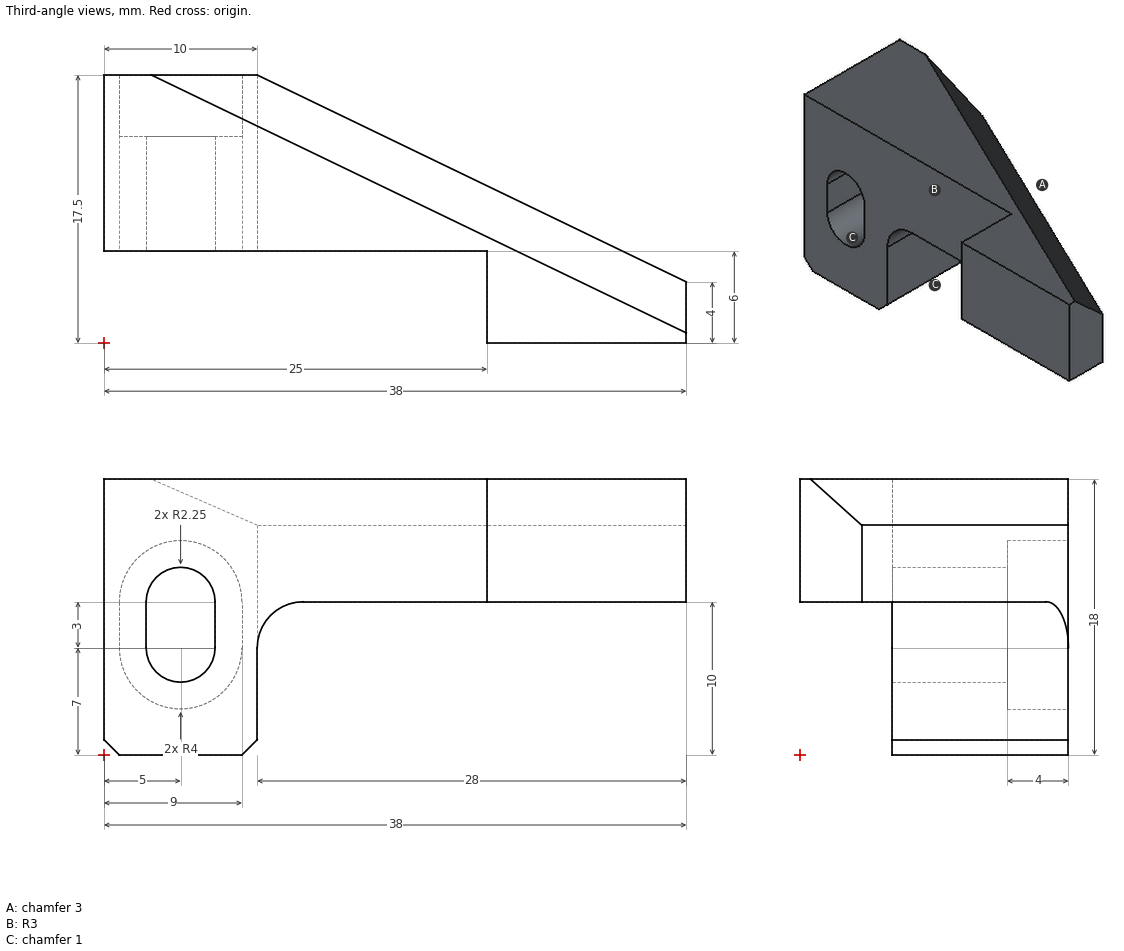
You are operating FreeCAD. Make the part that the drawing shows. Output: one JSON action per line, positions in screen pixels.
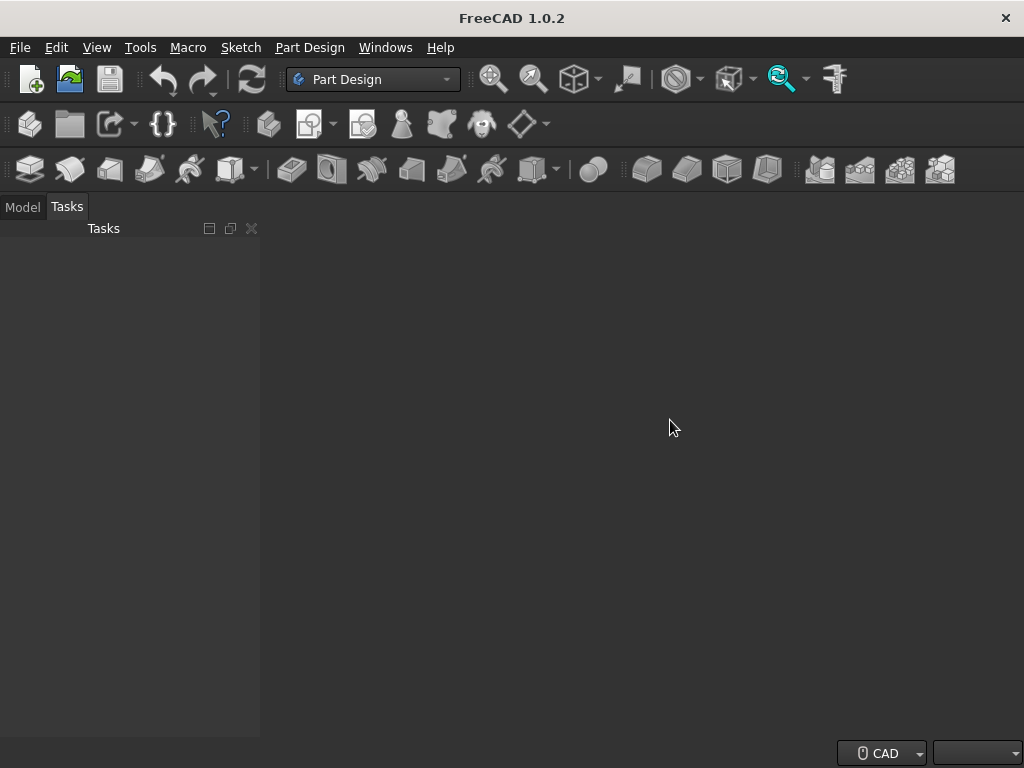
{"action": "key", "text": "ctrl+n"}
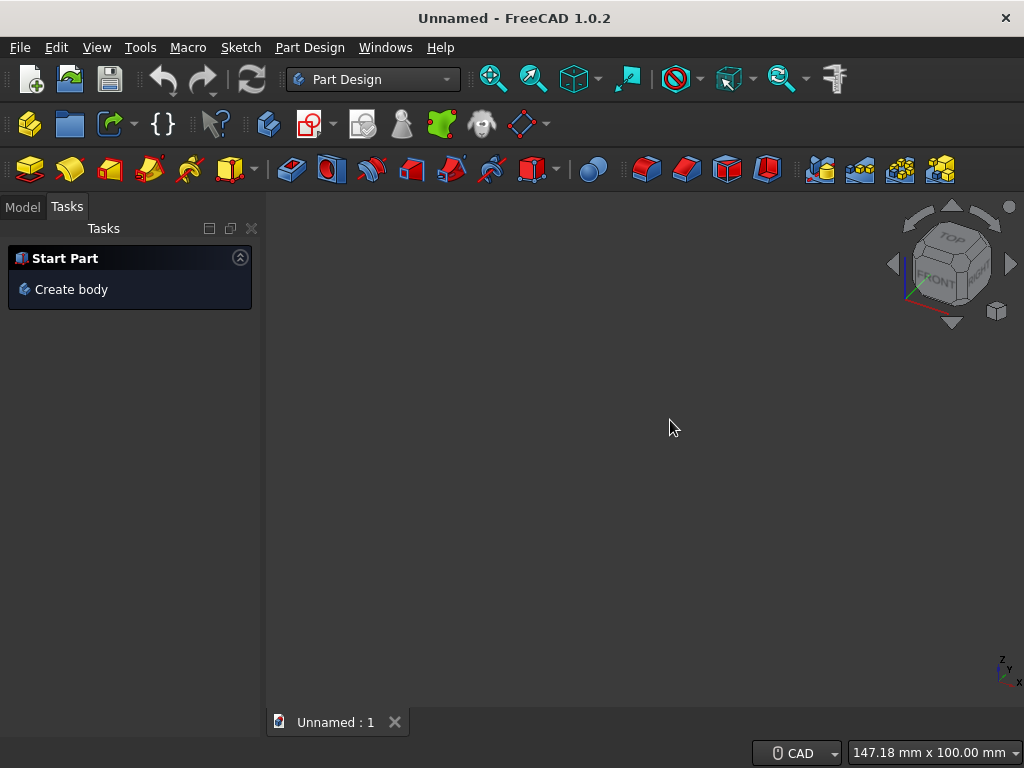
{"action": "left_click", "coordinate": [310, 124]}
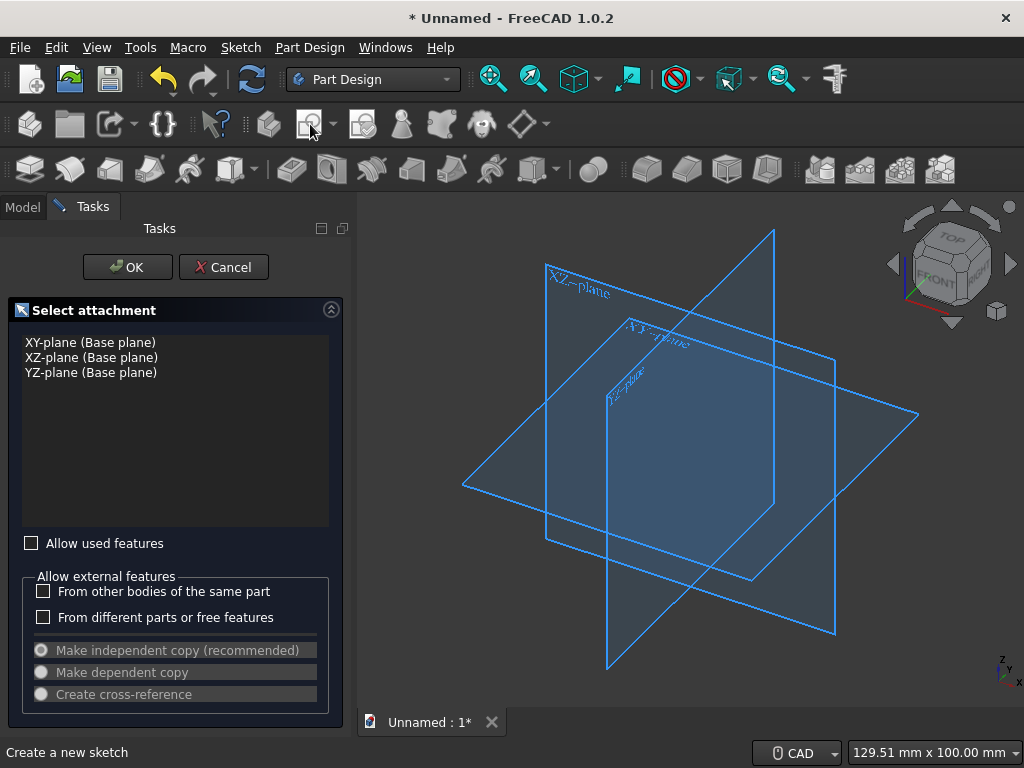
{"action": "left_click", "coordinate": [82, 342]}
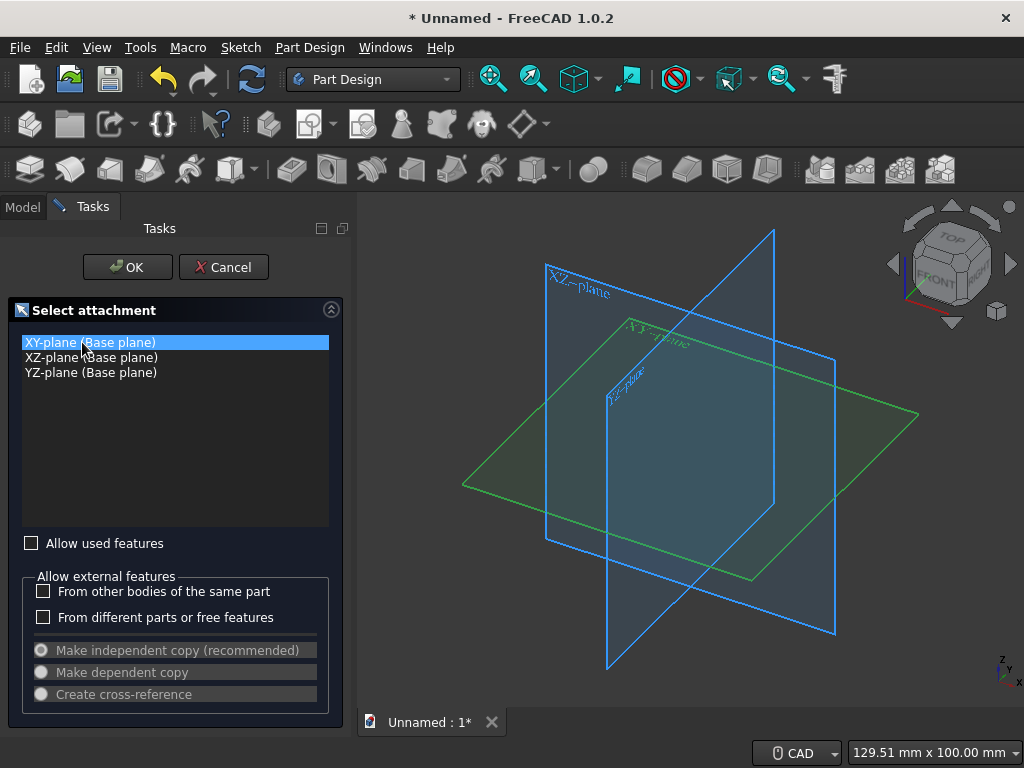
{"action": "left_click", "coordinate": [128, 267]}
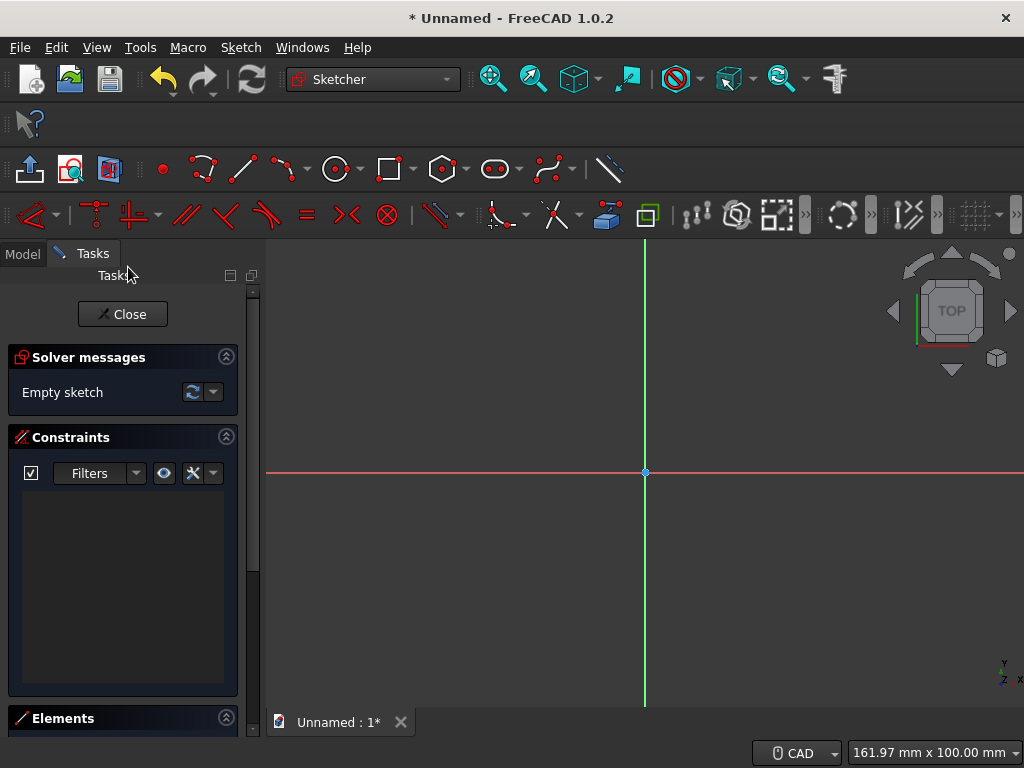
{"action": "scroll", "coordinate": [859, 399], "scroll_direction": "up", "scroll_amount": 4}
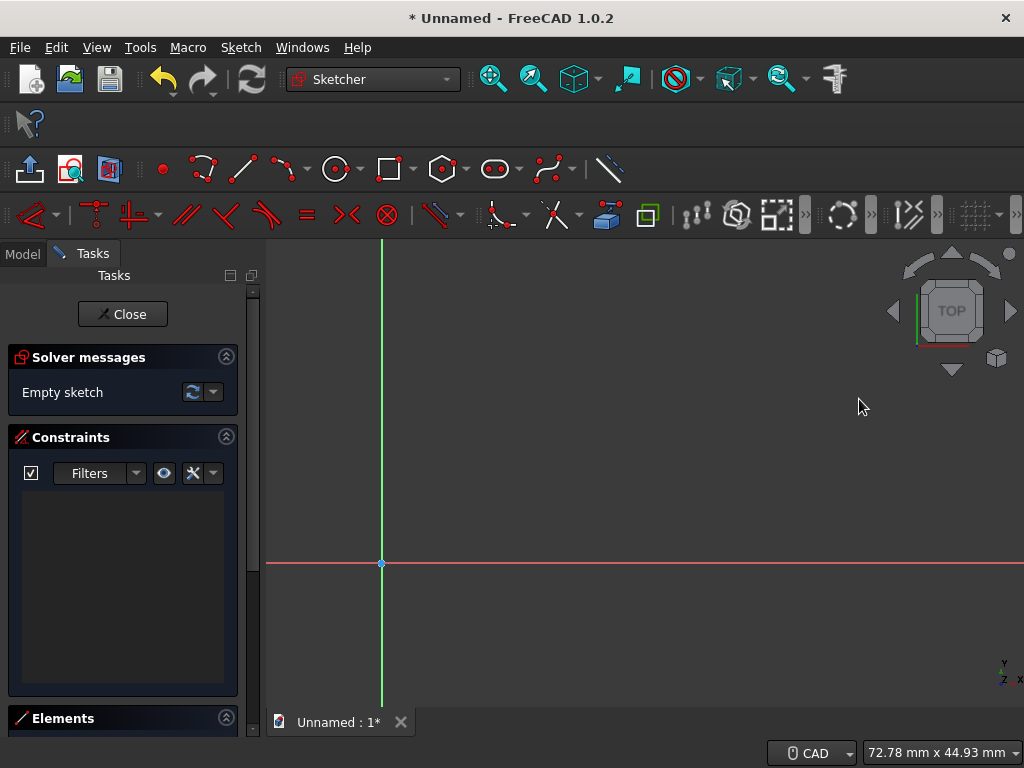
{"action": "key", "text": "g m"}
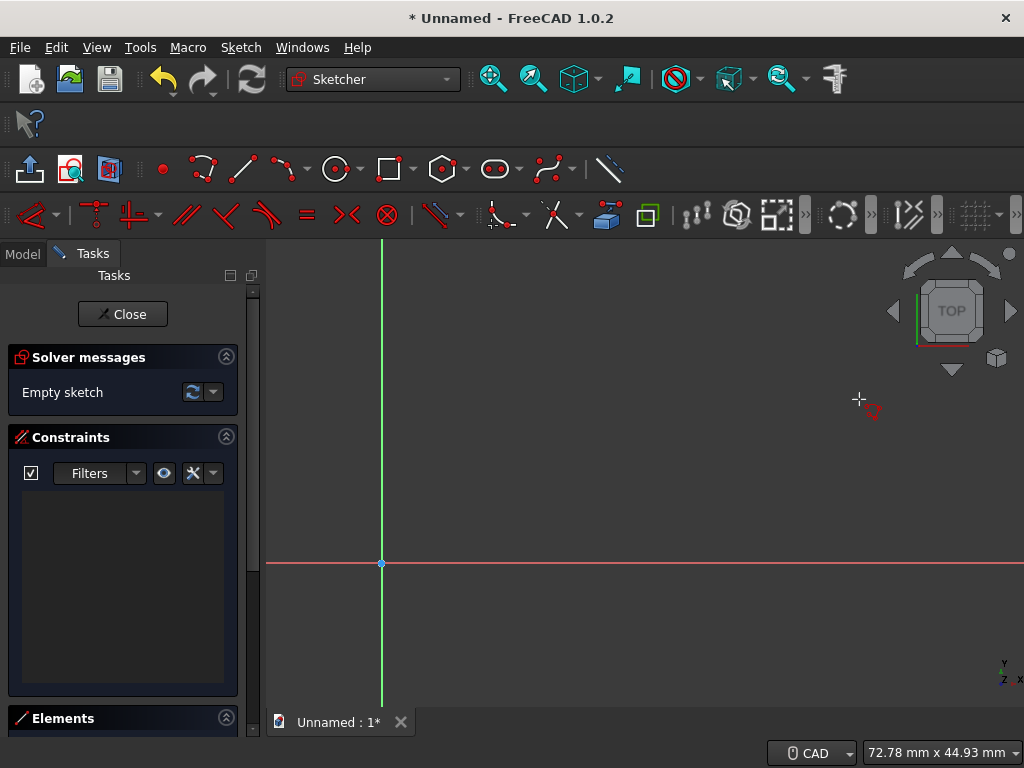
{"action": "left_click", "coordinate": [382, 563]}
{"action": "left_click", "coordinate": [778, 554]}
{"action": "left_click", "coordinate": [778, 522]}
{"action": "left_click", "coordinate": [486, 381]}
{"action": "left_click", "coordinate": [391, 381]}
{"action": "left_click", "coordinate": [382, 563]}
{"action": "key", "text": "Escape"}
{"action": "key", "text": "Escape"}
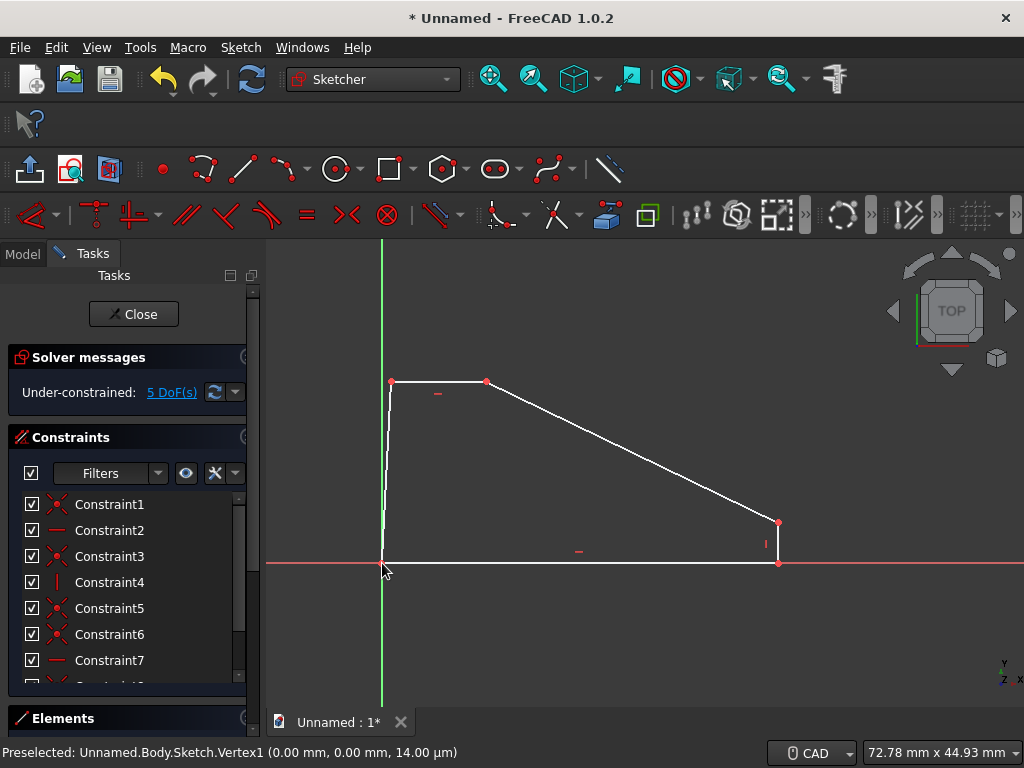
{"action": "left_click", "coordinate": [385, 509]}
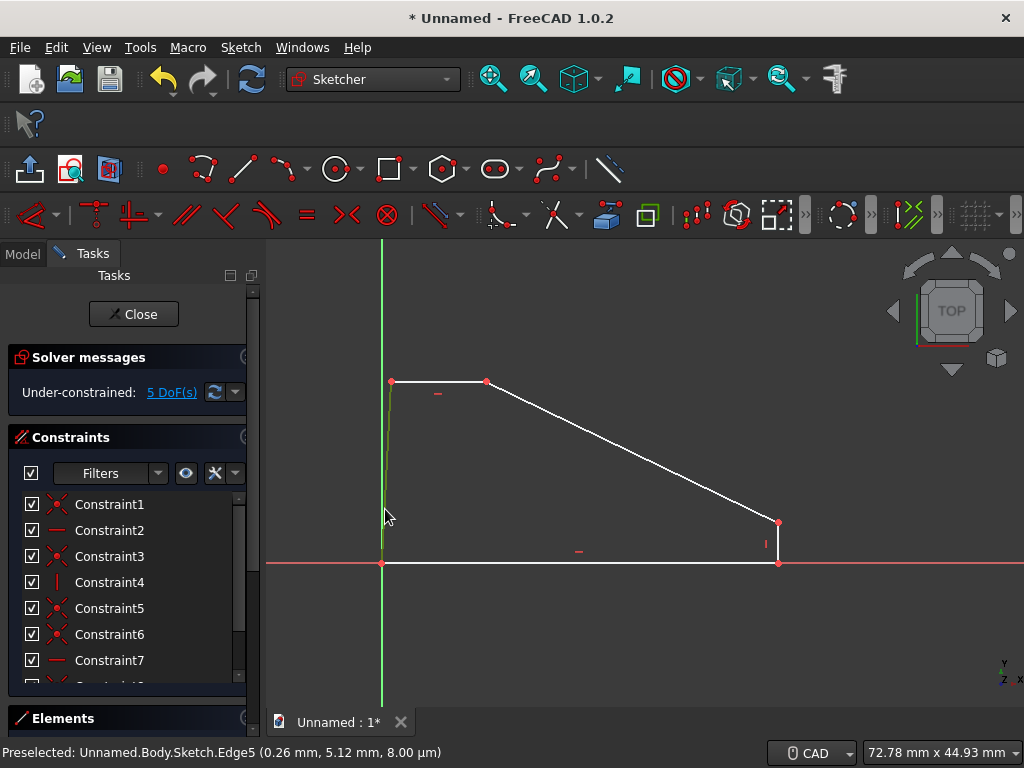
{"action": "key", "text": "v"}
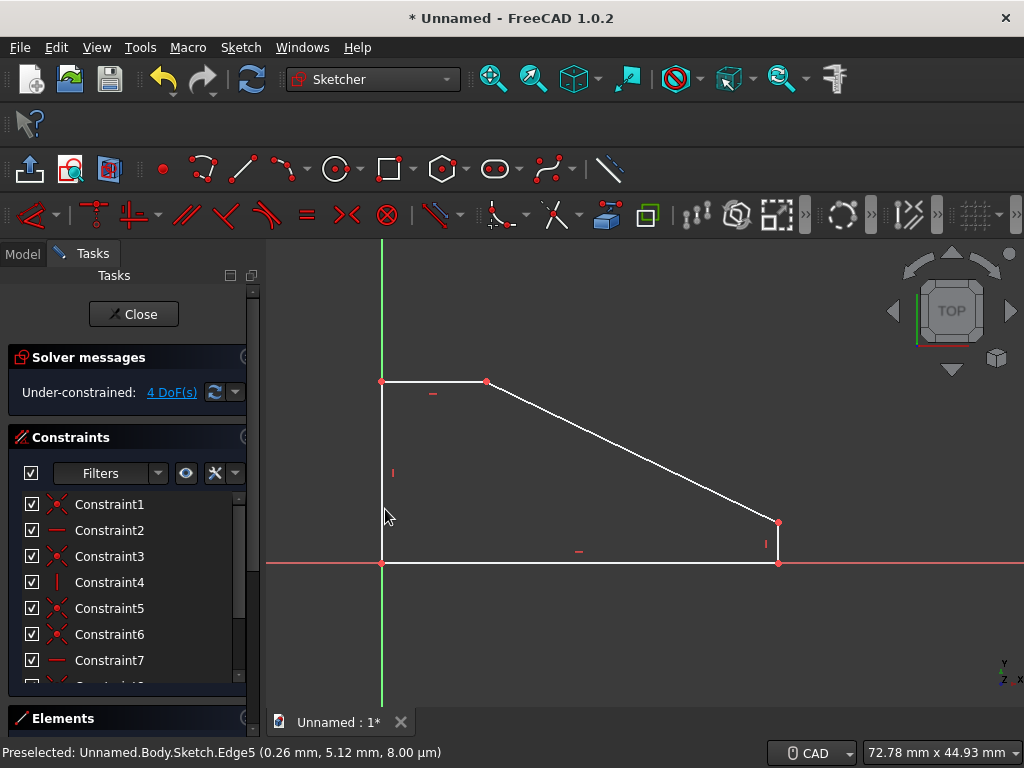
{"action": "left_click", "coordinate": [32, 216]}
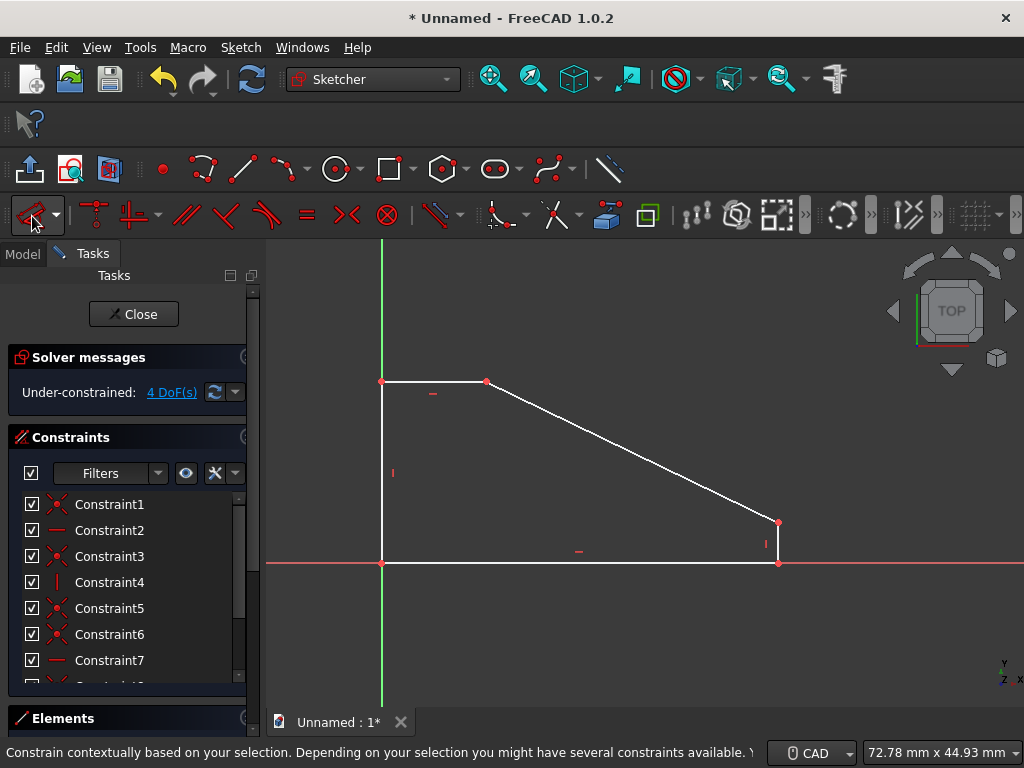
{"action": "left_click", "coordinate": [778, 551]}
{"action": "left_click", "coordinate": [812, 543]}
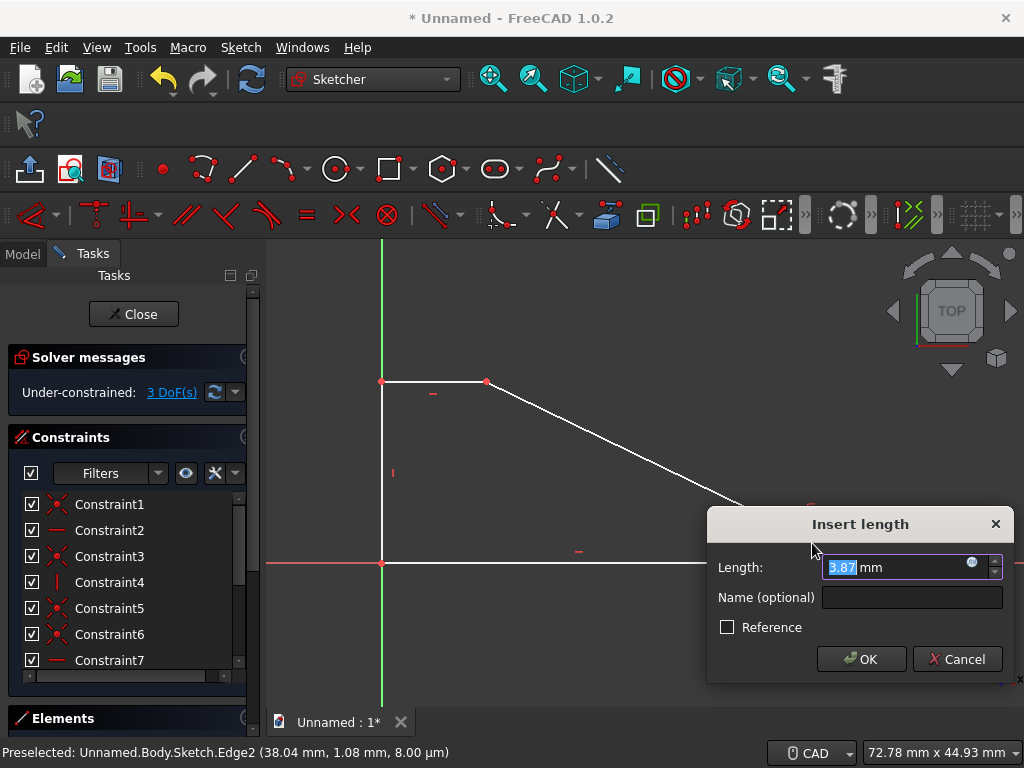
{"action": "type", "text": "4"}
{"action": "key", "text": "Return"}